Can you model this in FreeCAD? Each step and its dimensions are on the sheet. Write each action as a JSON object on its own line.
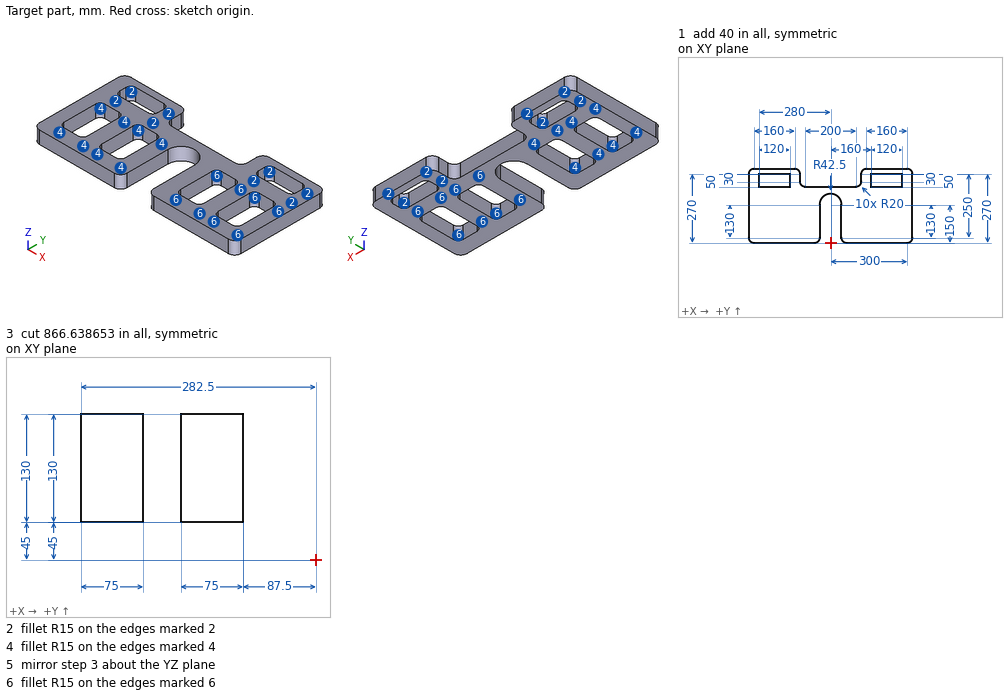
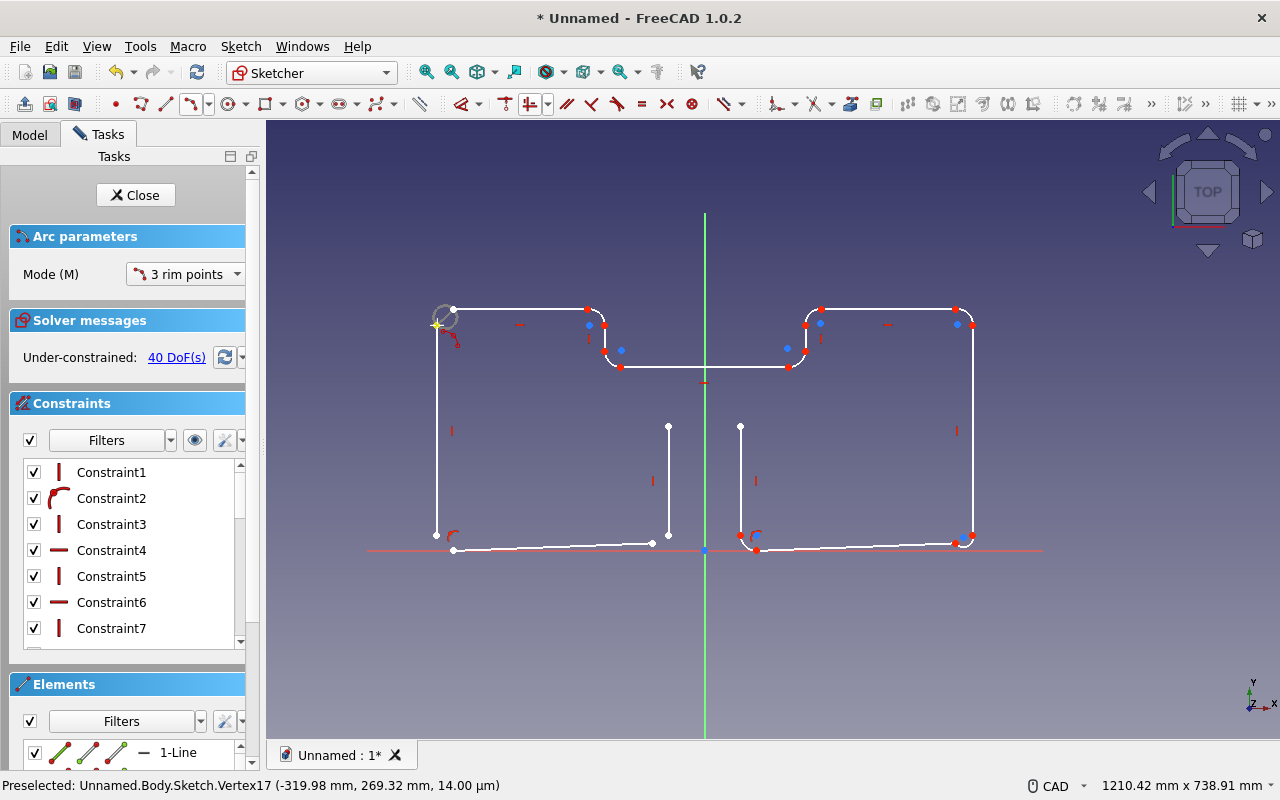
{"action": "scroll", "coordinate": [442, 313], "scroll_direction": "up", "scroll_amount": 6}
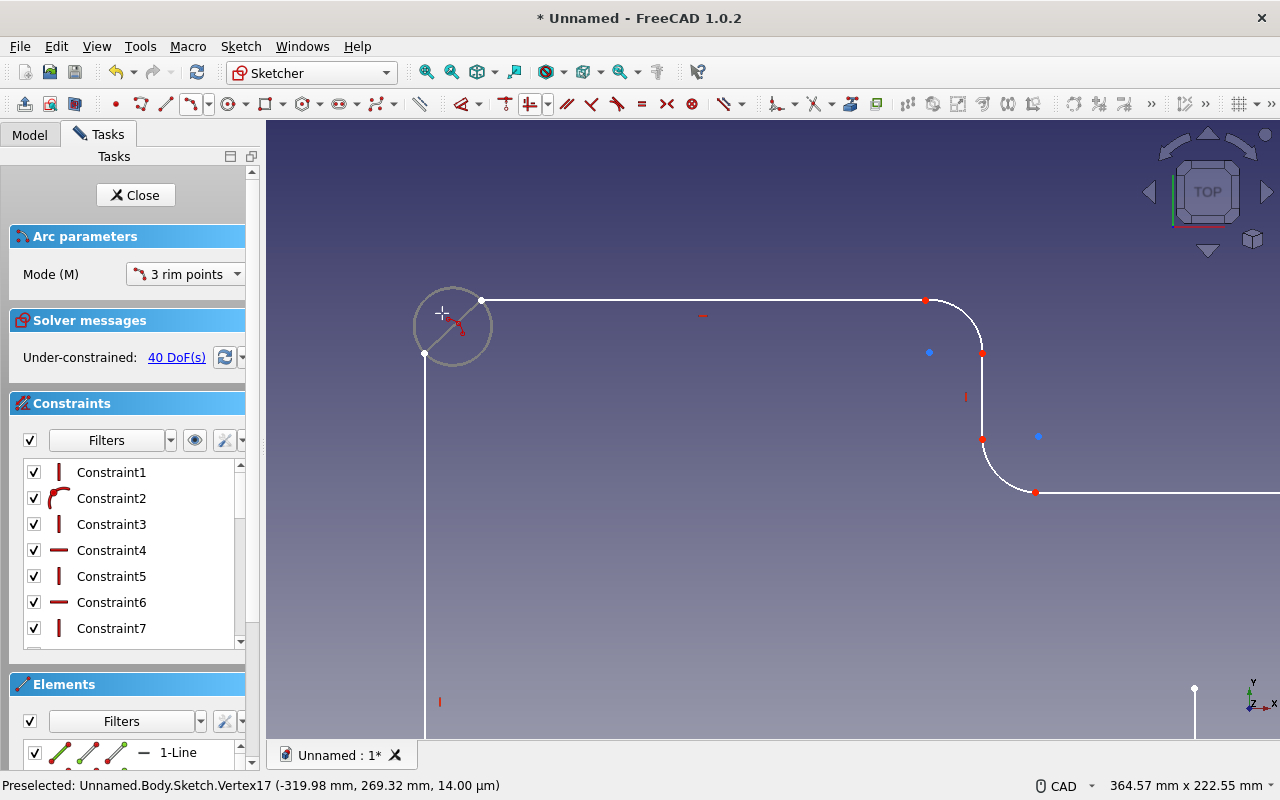
{"action": "left_click", "coordinate": [441, 312]}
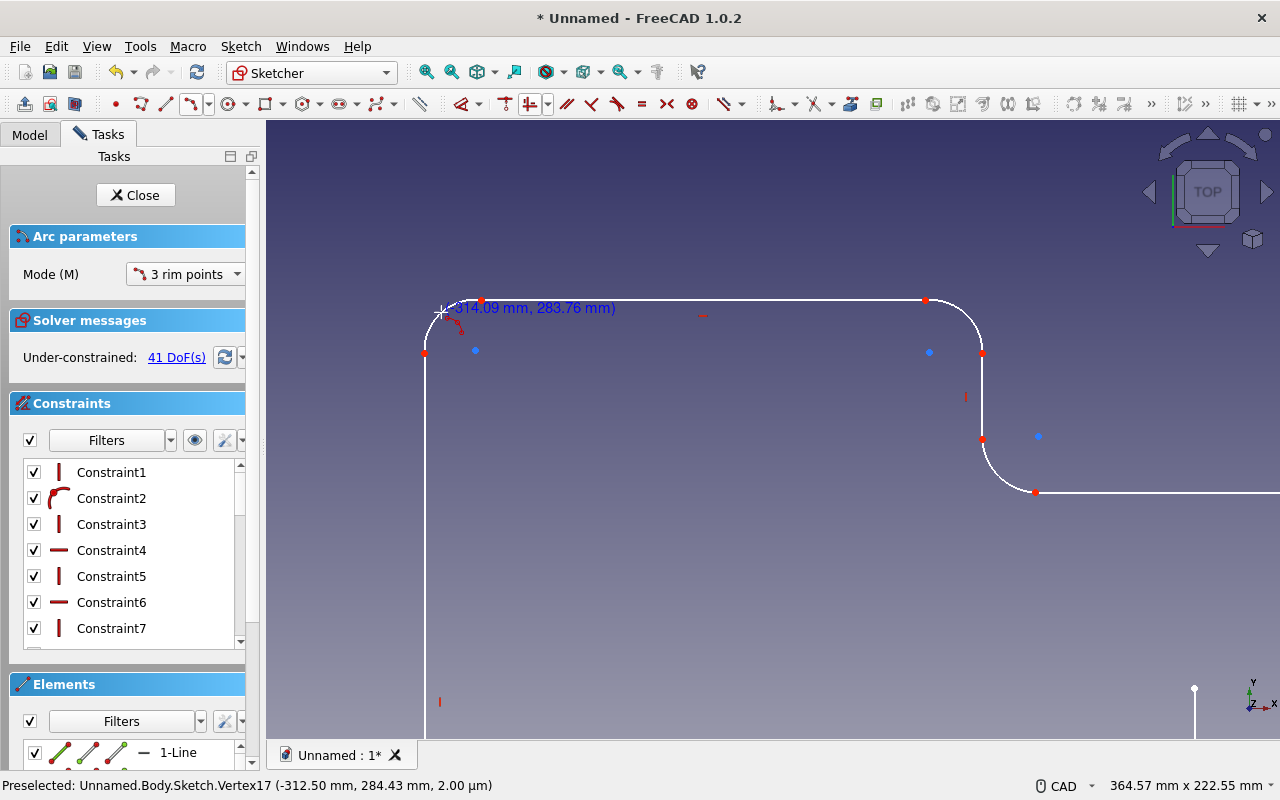
{"action": "scroll", "coordinate": [442, 313], "scroll_direction": "down", "scroll_amount": 6}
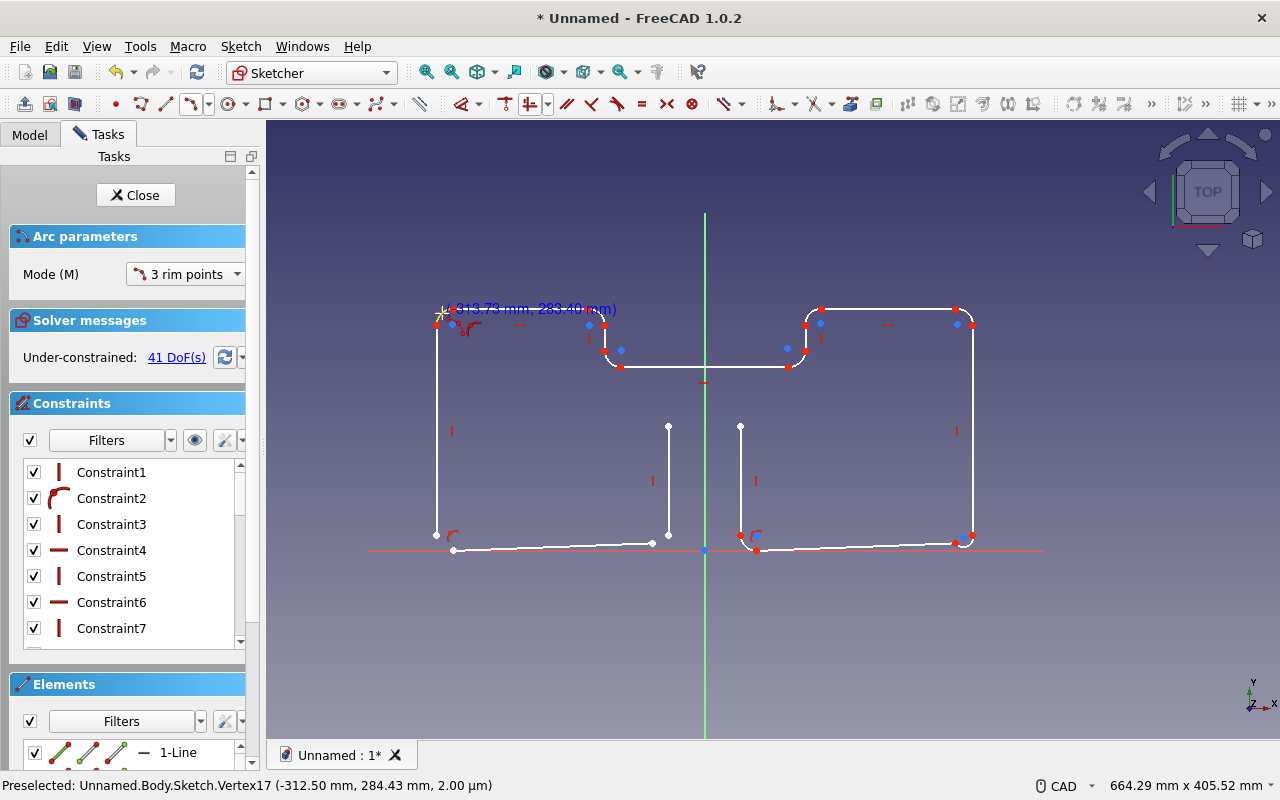
{"action": "left_click", "coordinate": [437, 535]}
{"action": "left_click", "coordinate": [454, 551]}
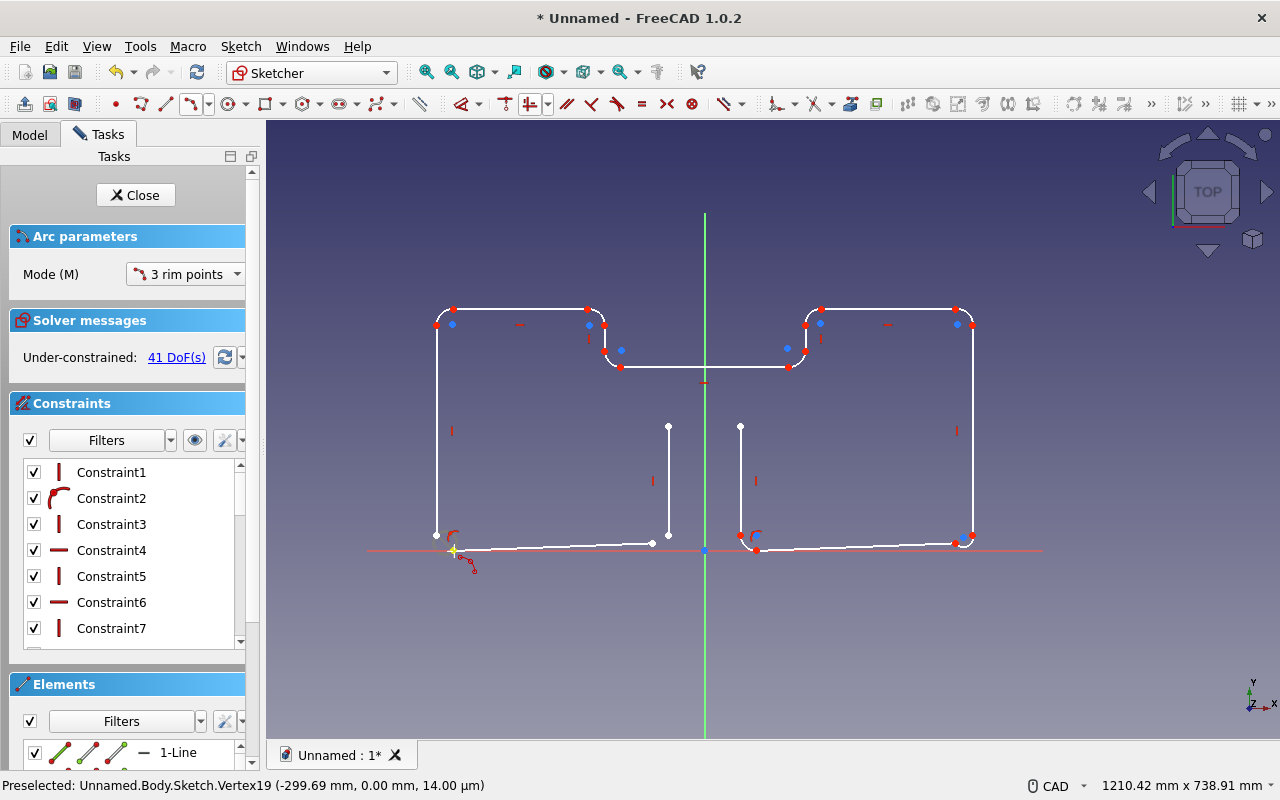
{"action": "scroll", "coordinate": [442, 546], "scroll_direction": "up", "scroll_amount": 6}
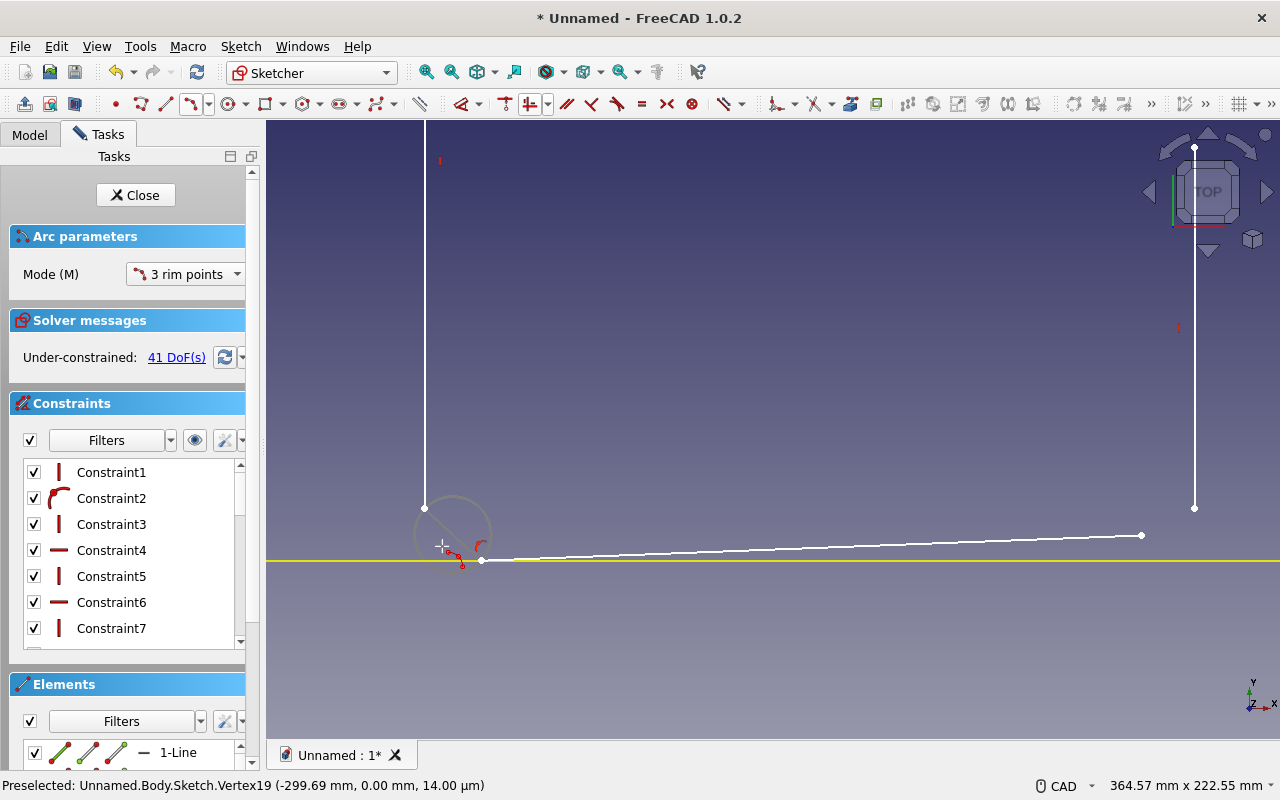
{"action": "left_click", "coordinate": [441, 544]}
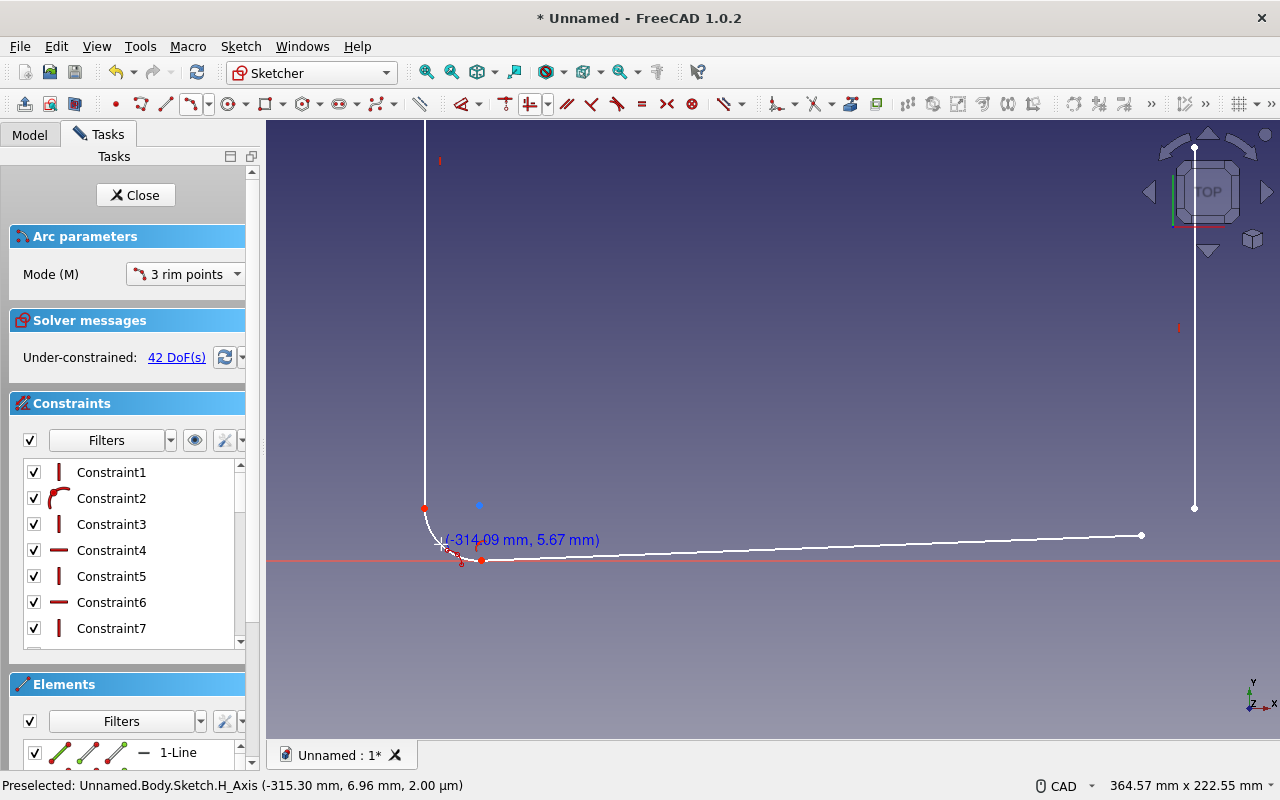
{"action": "scroll", "coordinate": [442, 547], "scroll_direction": "down", "scroll_amount": 6}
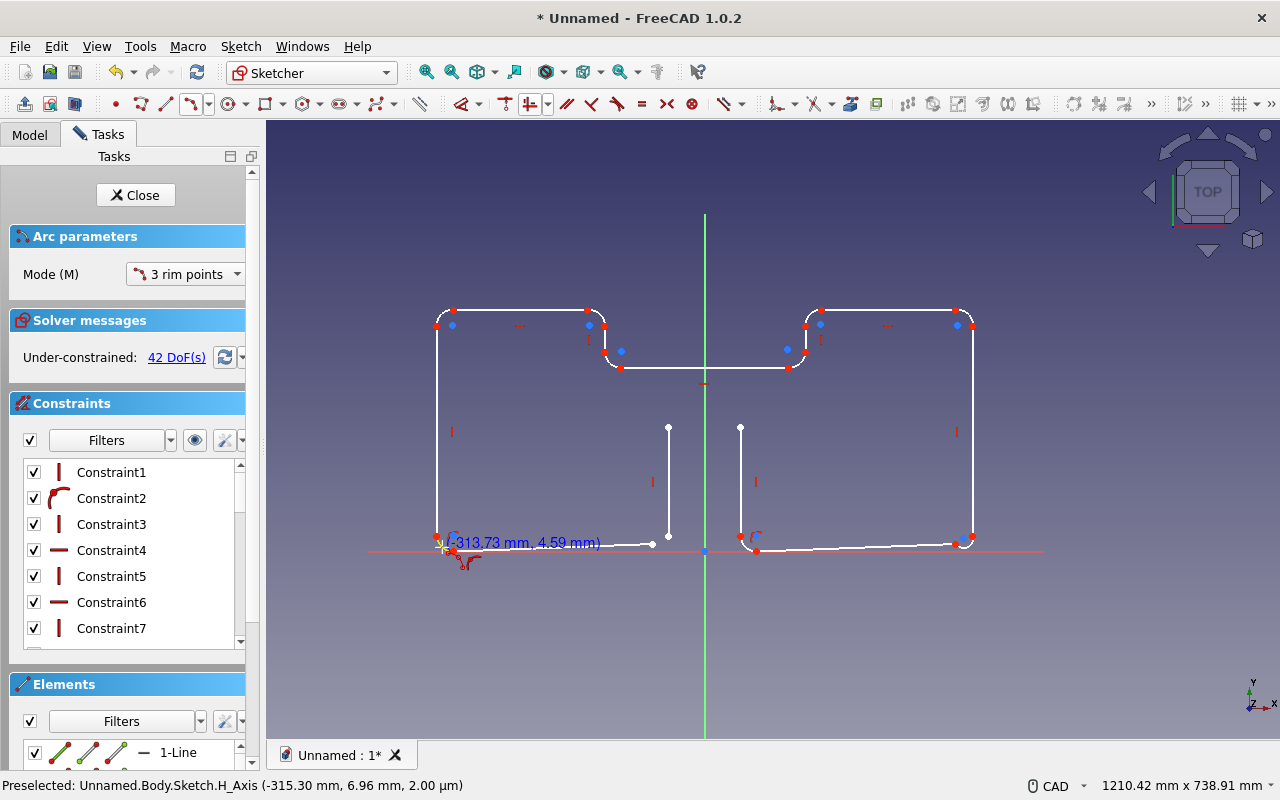
{"action": "left_click", "coordinate": [653, 544]}
{"action": "left_click", "coordinate": [669, 536]}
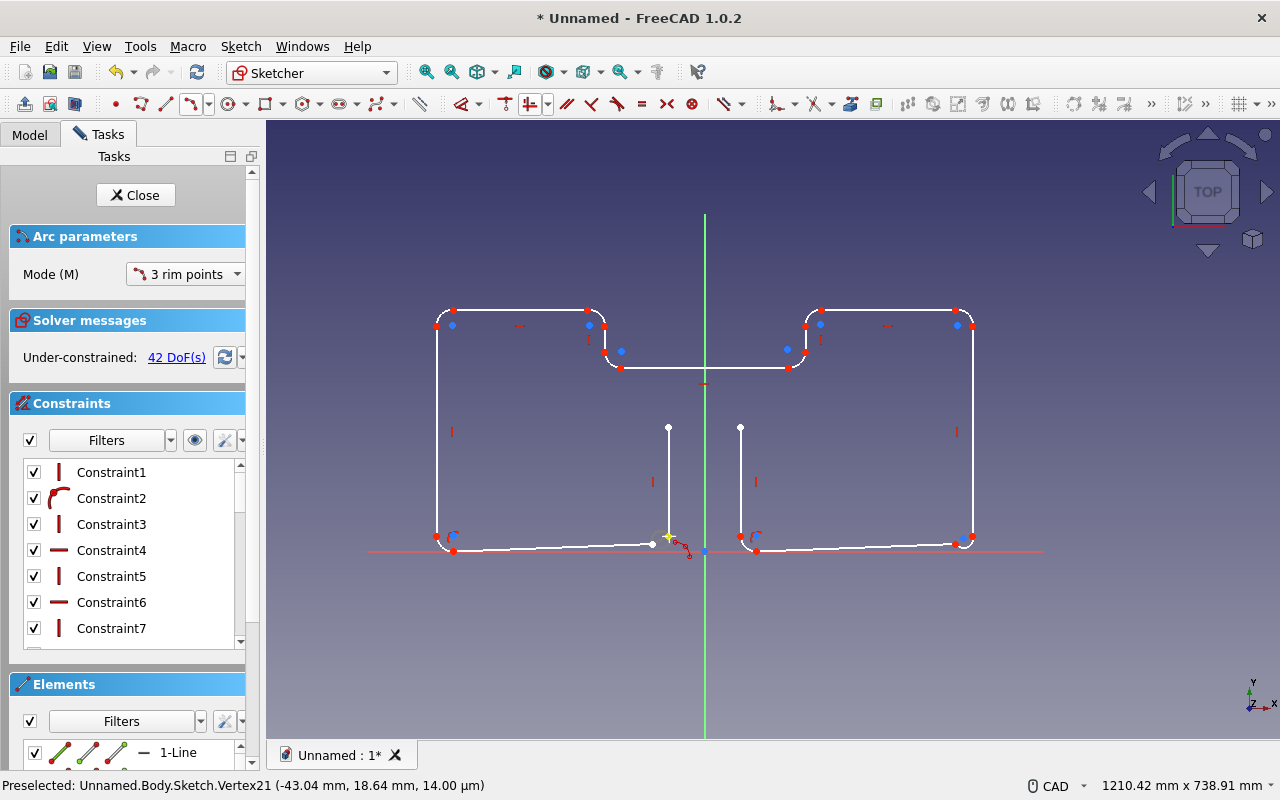
{"action": "scroll", "coordinate": [664, 547], "scroll_direction": "up", "scroll_amount": 6}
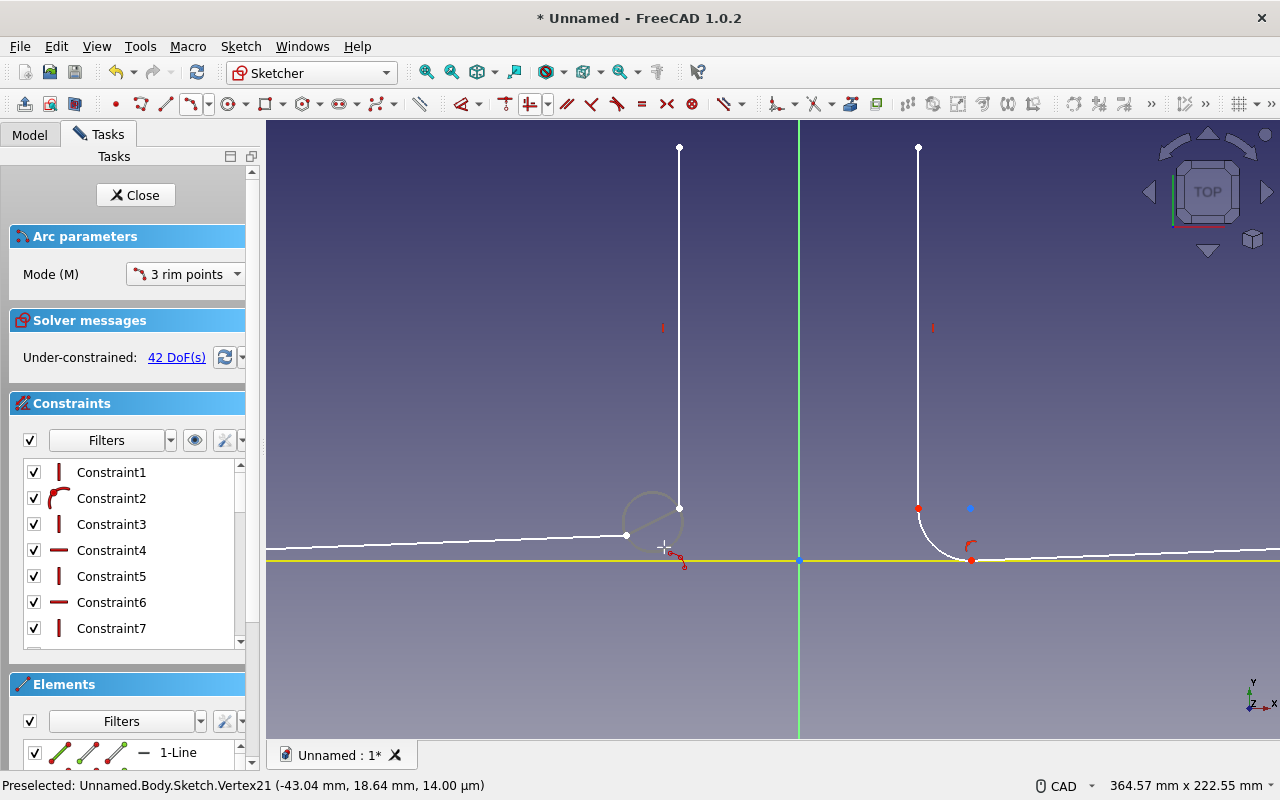
{"action": "left_click", "coordinate": [665, 544]}